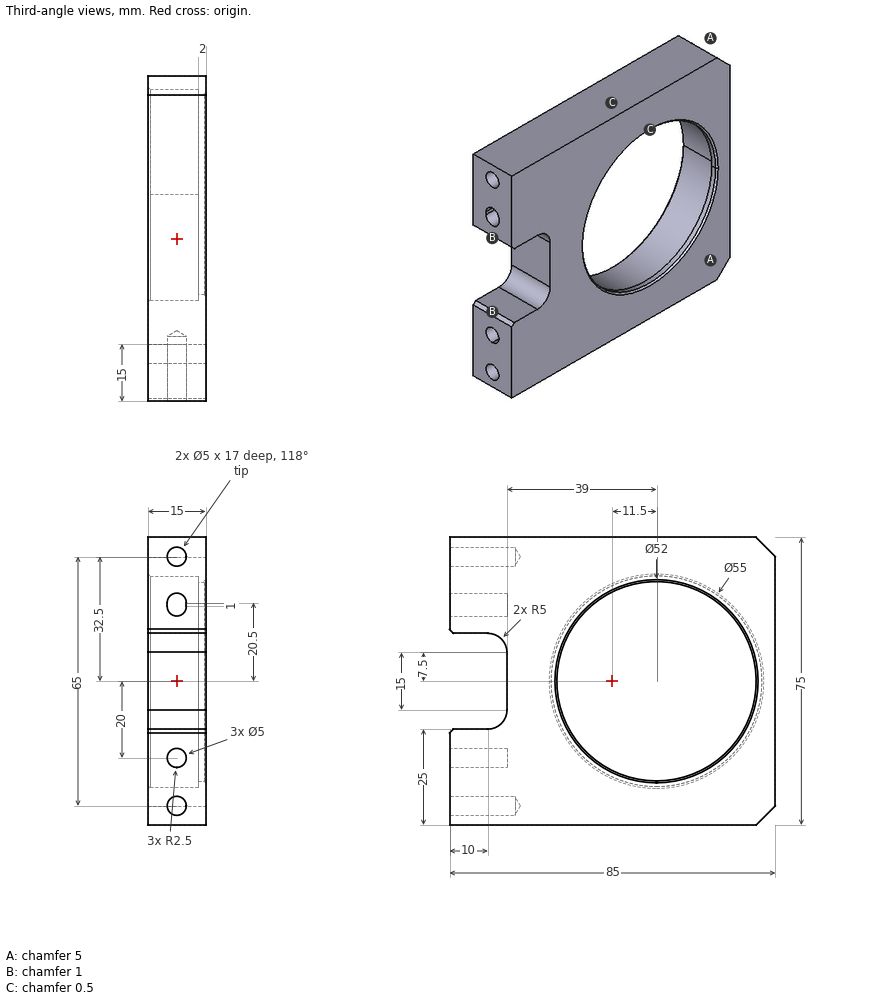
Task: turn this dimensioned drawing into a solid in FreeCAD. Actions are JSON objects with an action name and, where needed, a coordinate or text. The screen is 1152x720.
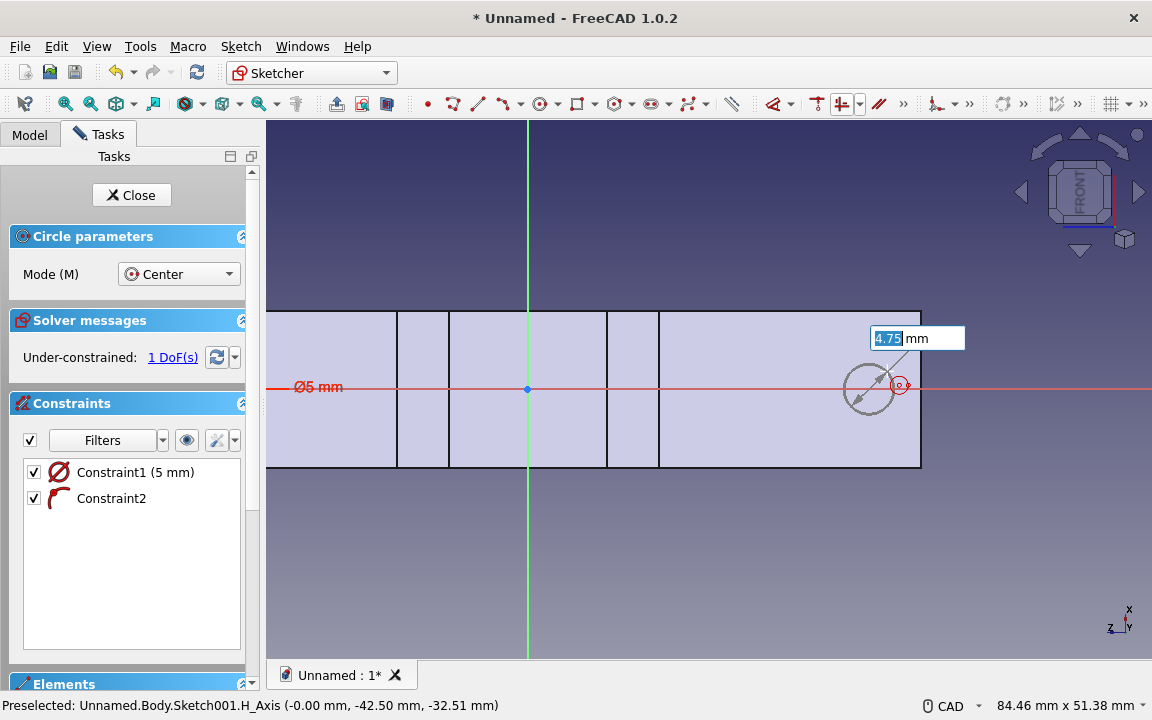
{"action": "type", "text": "5"}
{"action": "key", "text": "Return"}
{"action": "key", "text": "Escape"}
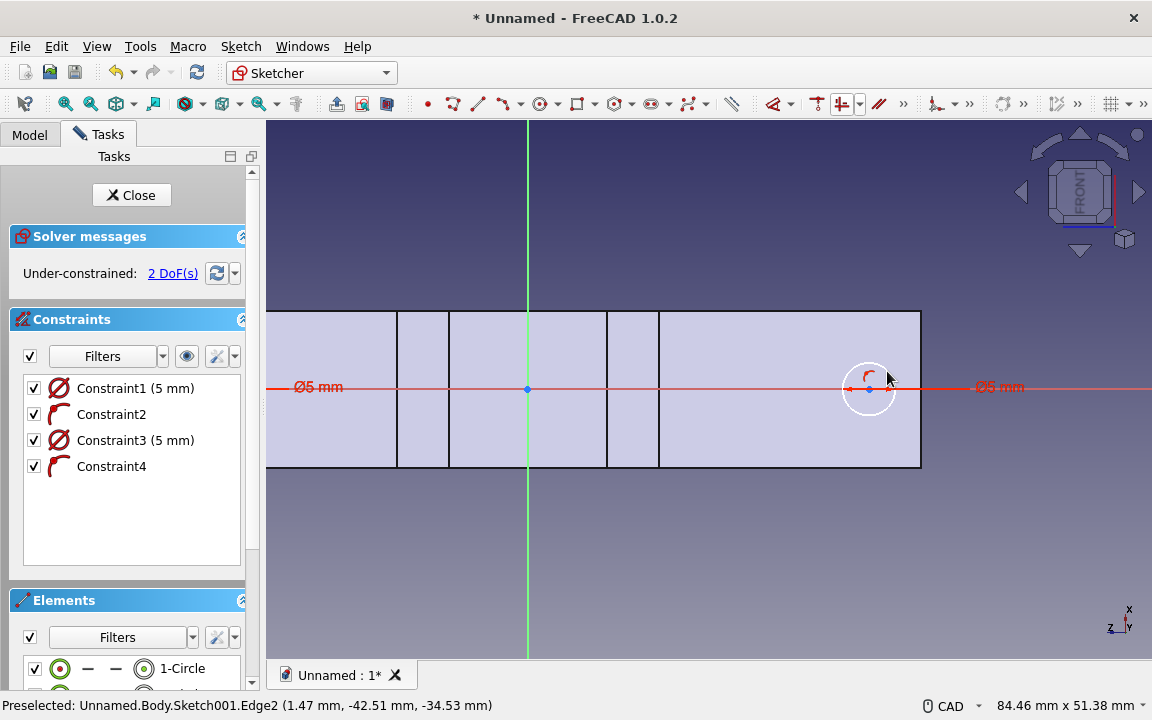
{"action": "left_click", "coordinate": [772, 104]}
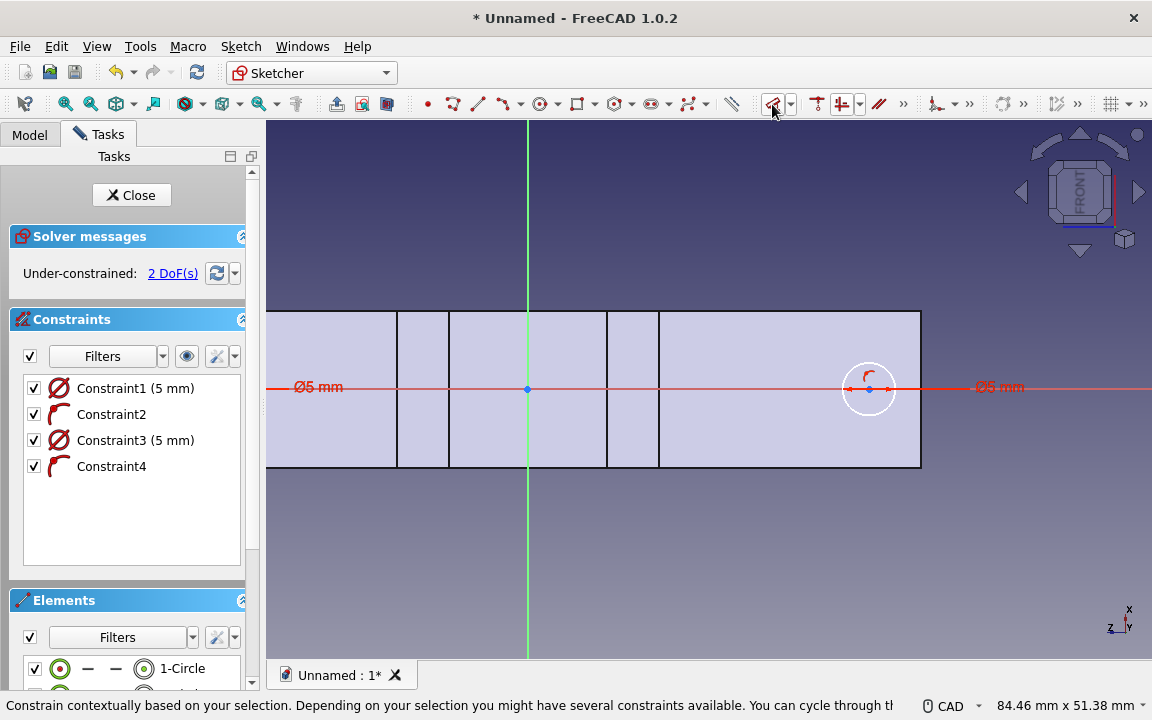
{"action": "scroll", "coordinate": [869, 390], "scroll_direction": "down", "scroll_amount": 2}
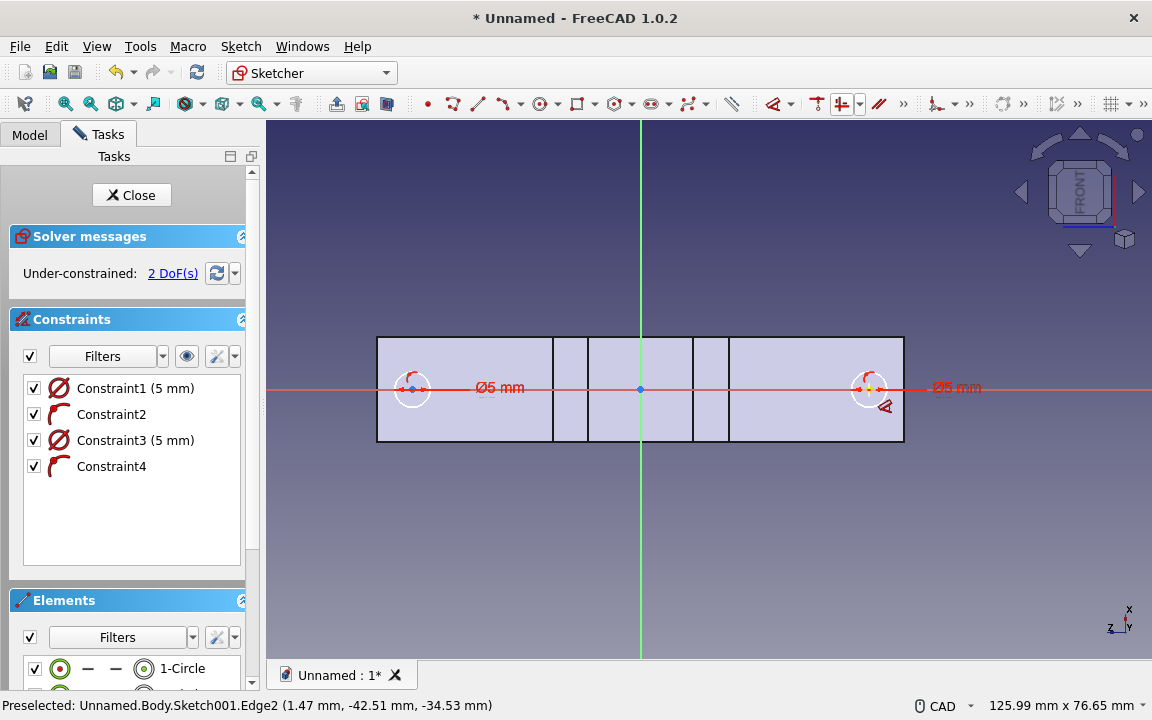
{"action": "left_click", "coordinate": [412, 390]}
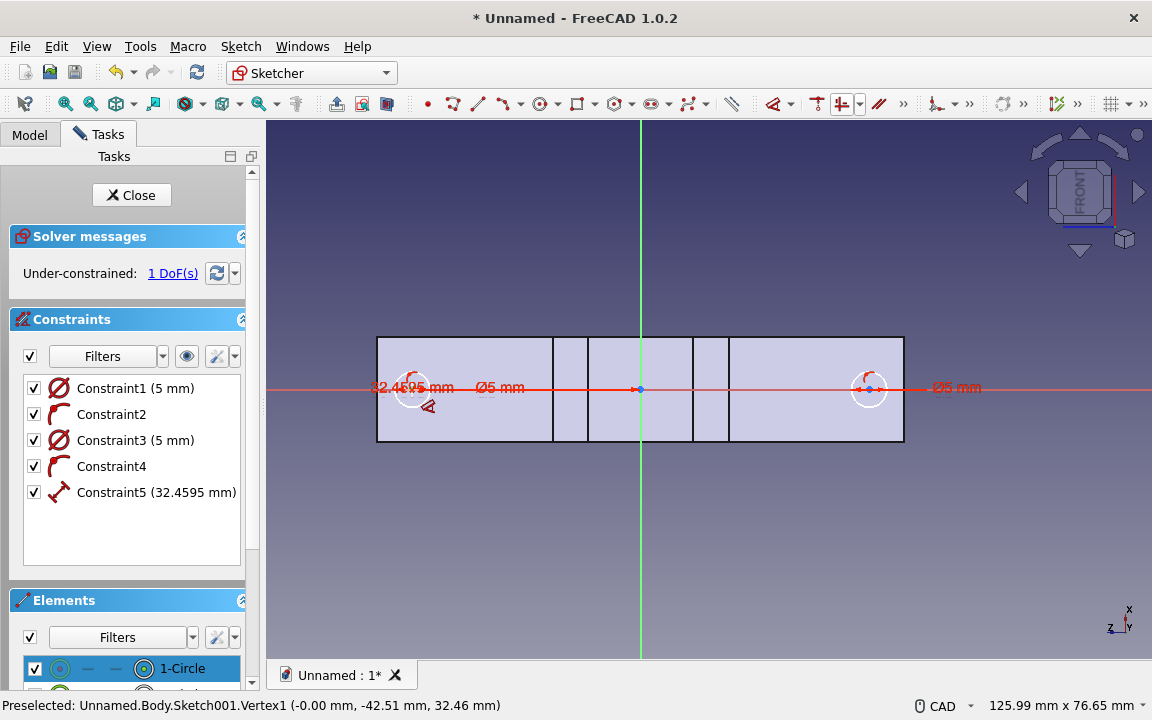
{"action": "left_click", "coordinate": [869, 390]}
{"action": "left_click", "coordinate": [536, 424]}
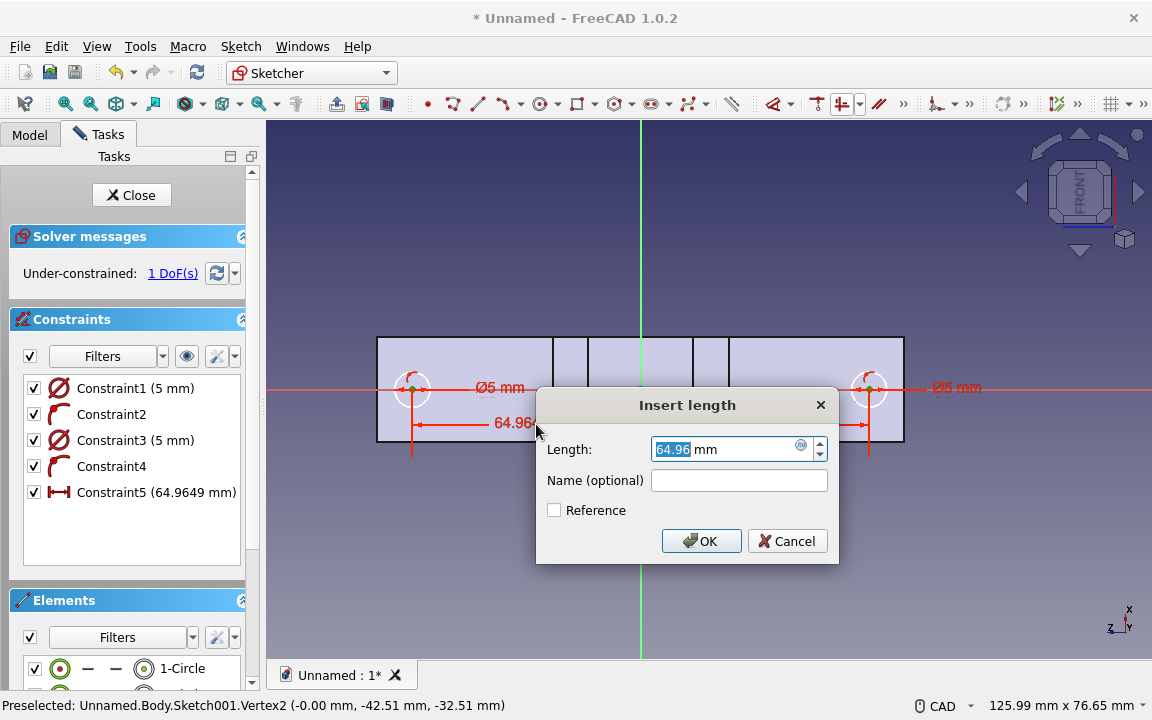
{"action": "type", "text": "65"}
{"action": "key", "text": "Return"}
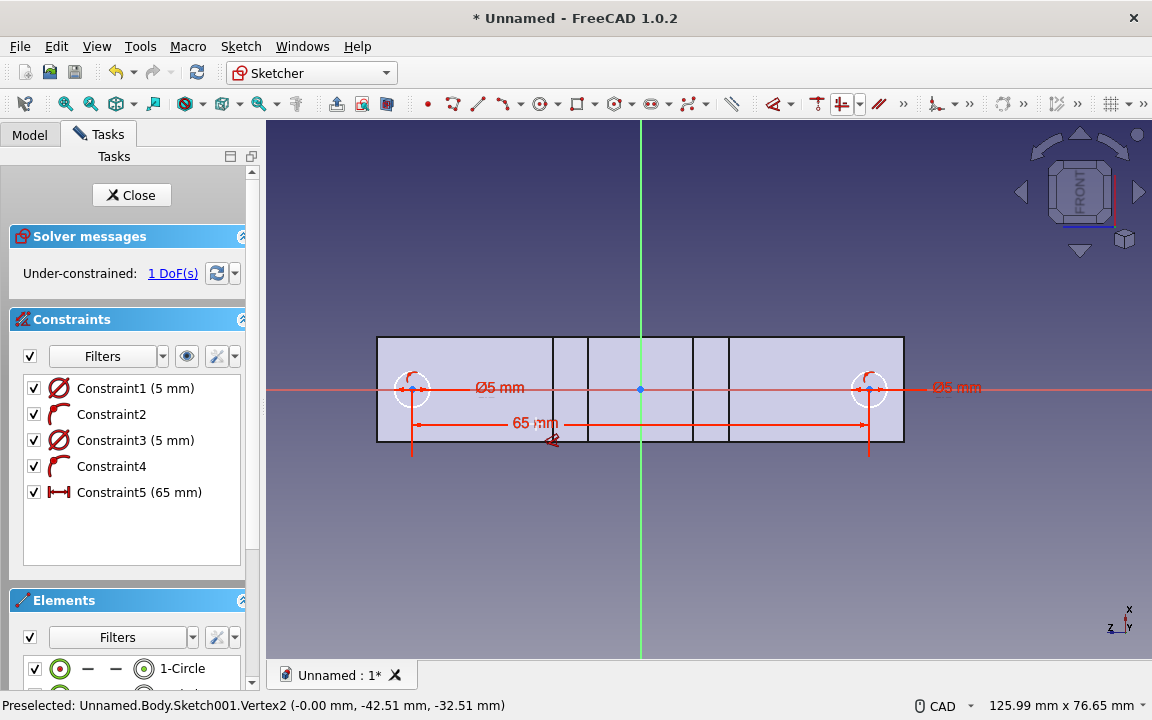
{"action": "left_click", "coordinate": [412, 390]}
{"action": "left_click", "coordinate": [446, 424]}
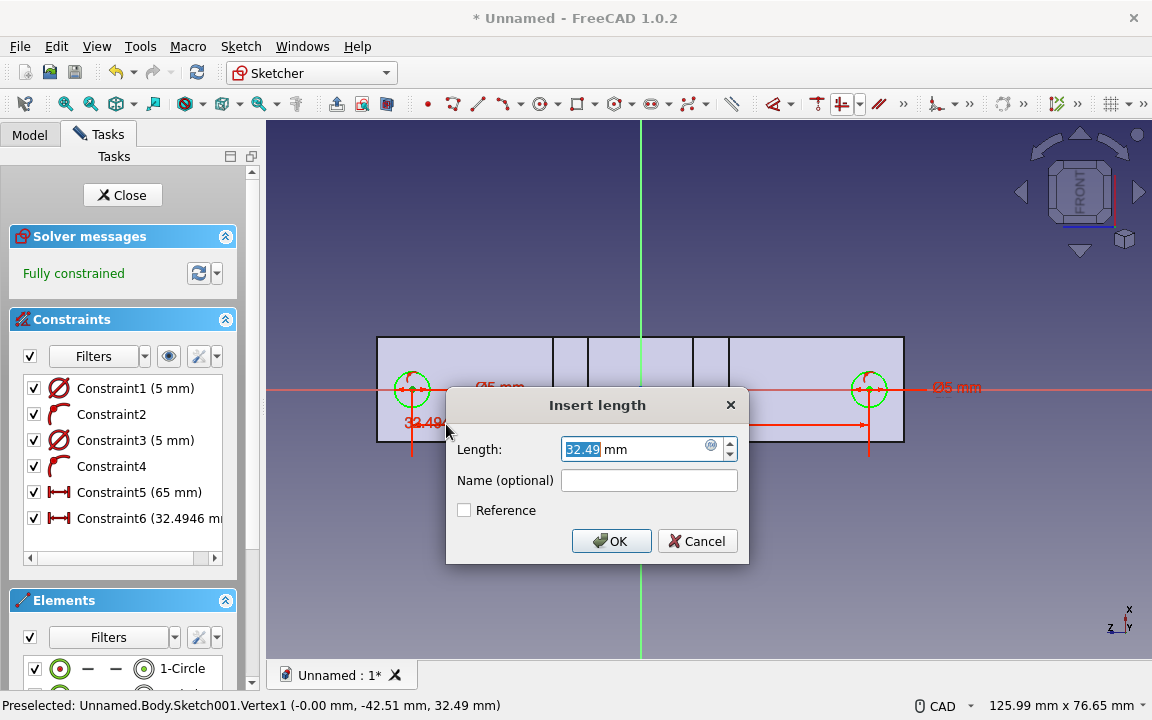
{"action": "type", "text": "32.5"}
{"action": "key", "text": "Return"}
{"action": "key", "text": "Escape"}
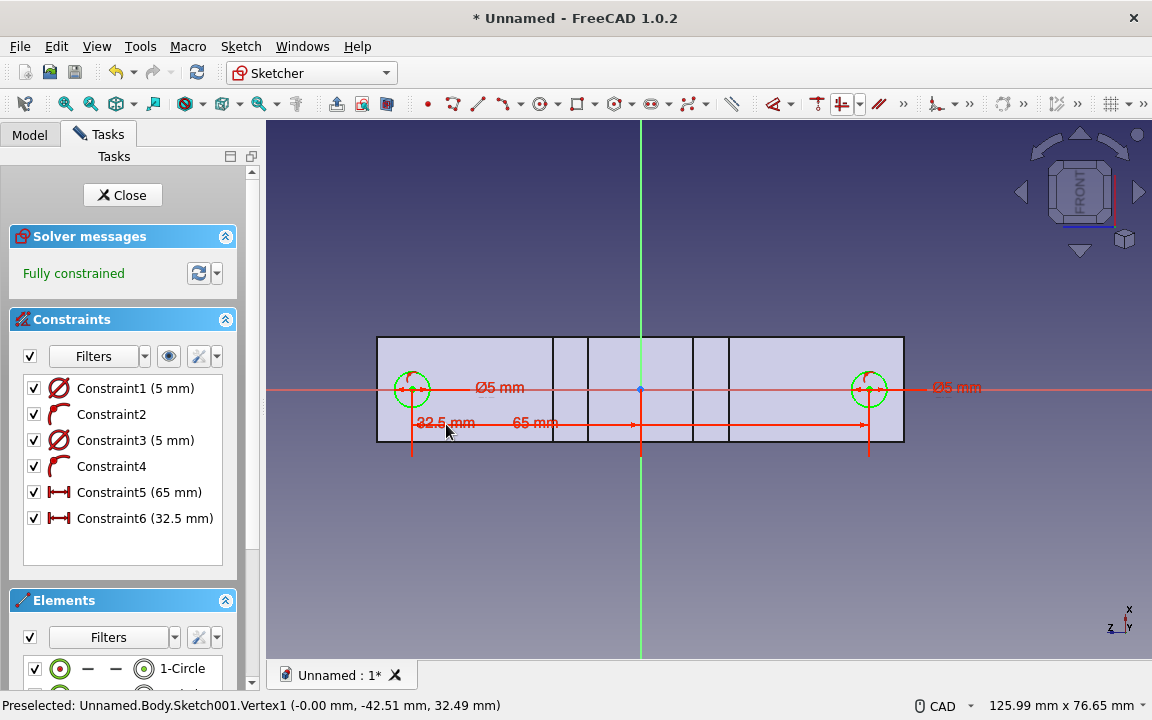
{"action": "left_click", "coordinate": [123, 195]}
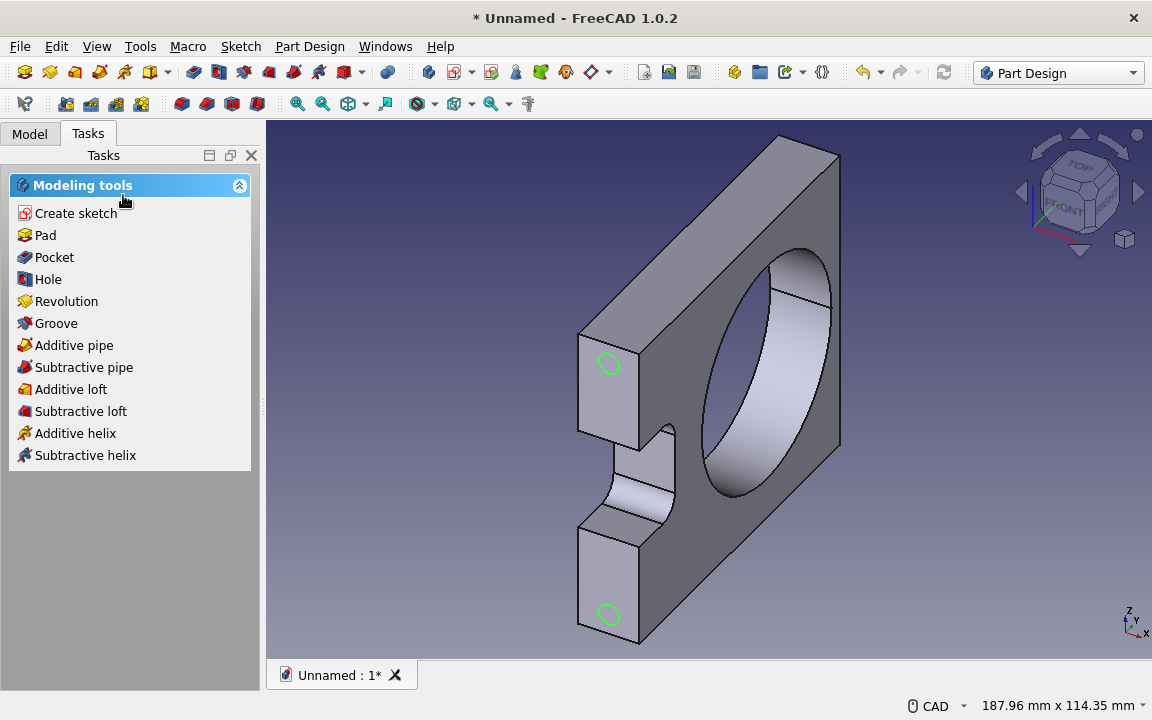
{"action": "left_click", "coordinate": [219, 72]}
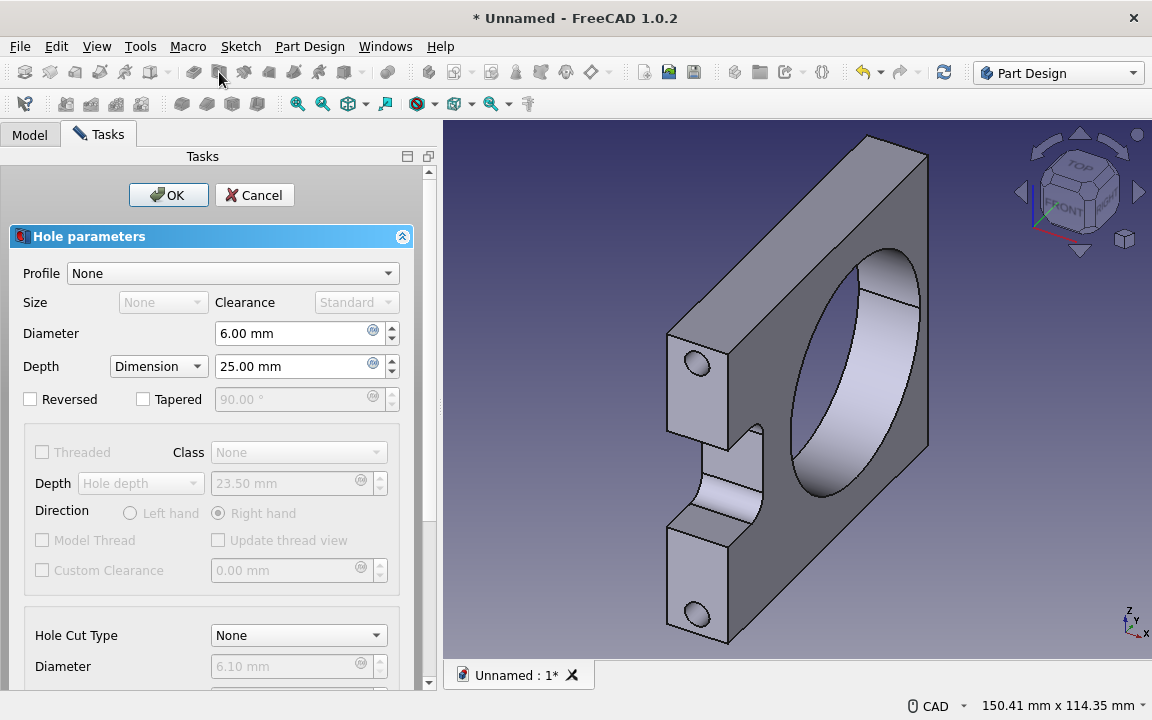
{"action": "triple_click", "coordinate": [300, 334]}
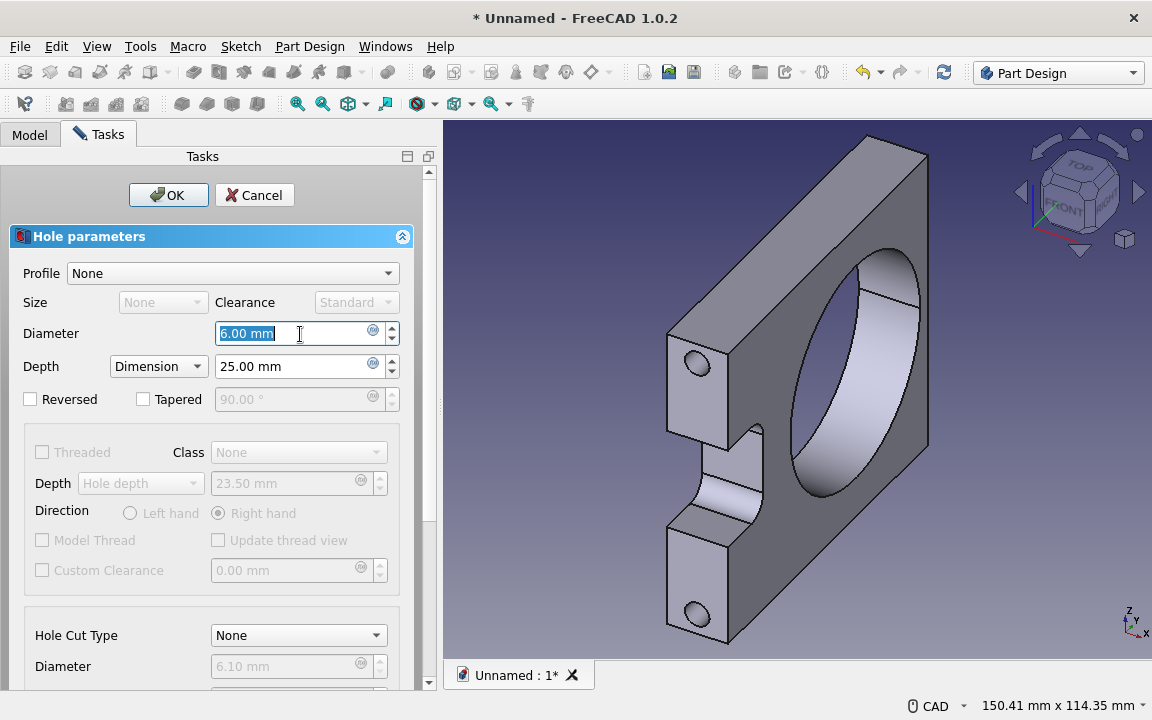
{"action": "type", "text": "5"}
{"action": "key", "text": "Tab"}